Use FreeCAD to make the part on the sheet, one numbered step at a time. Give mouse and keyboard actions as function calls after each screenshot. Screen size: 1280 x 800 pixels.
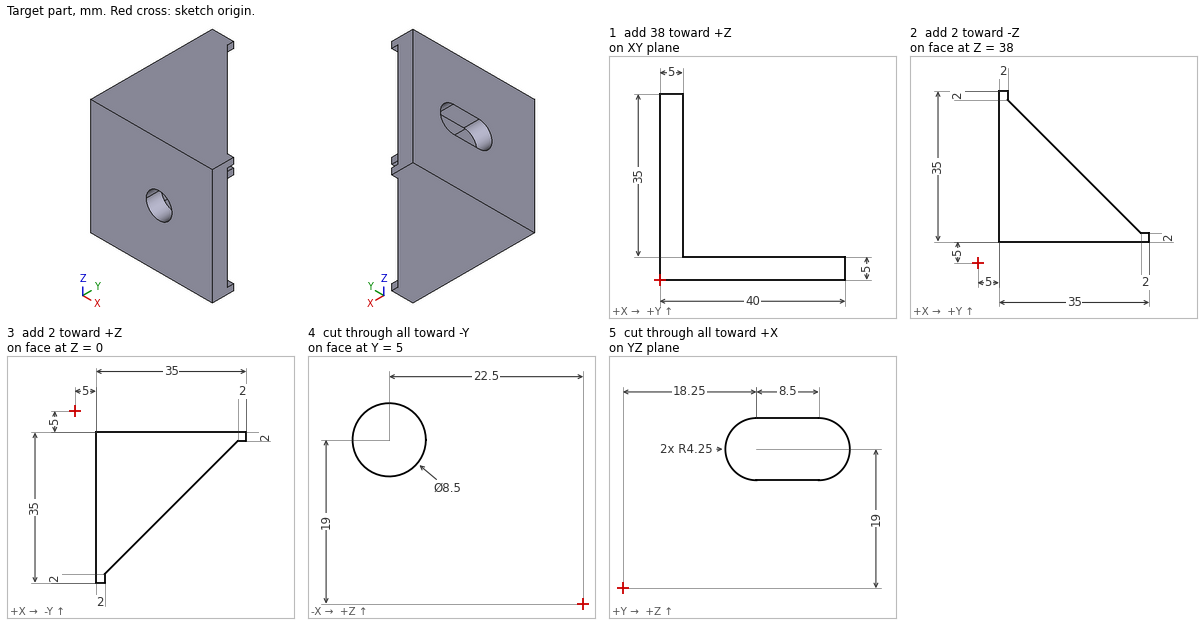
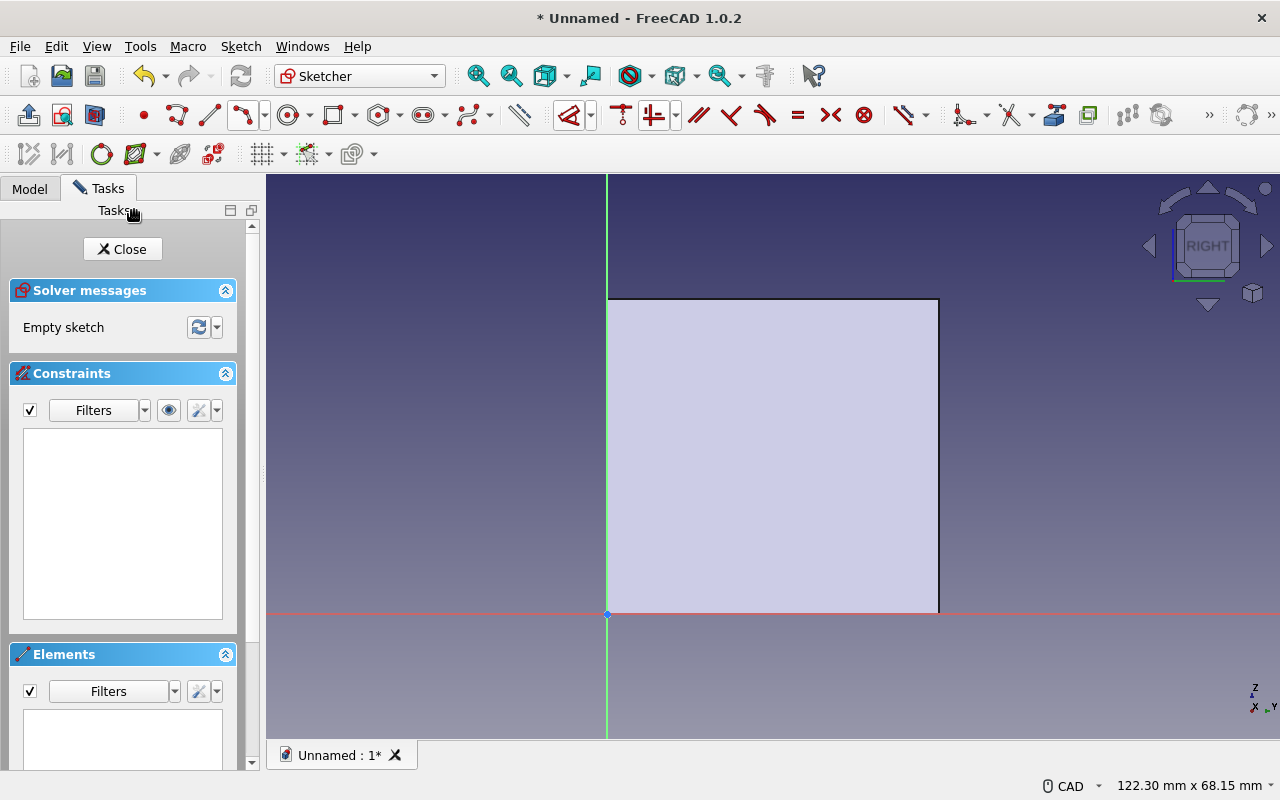
scroll(774, 592, up, 3)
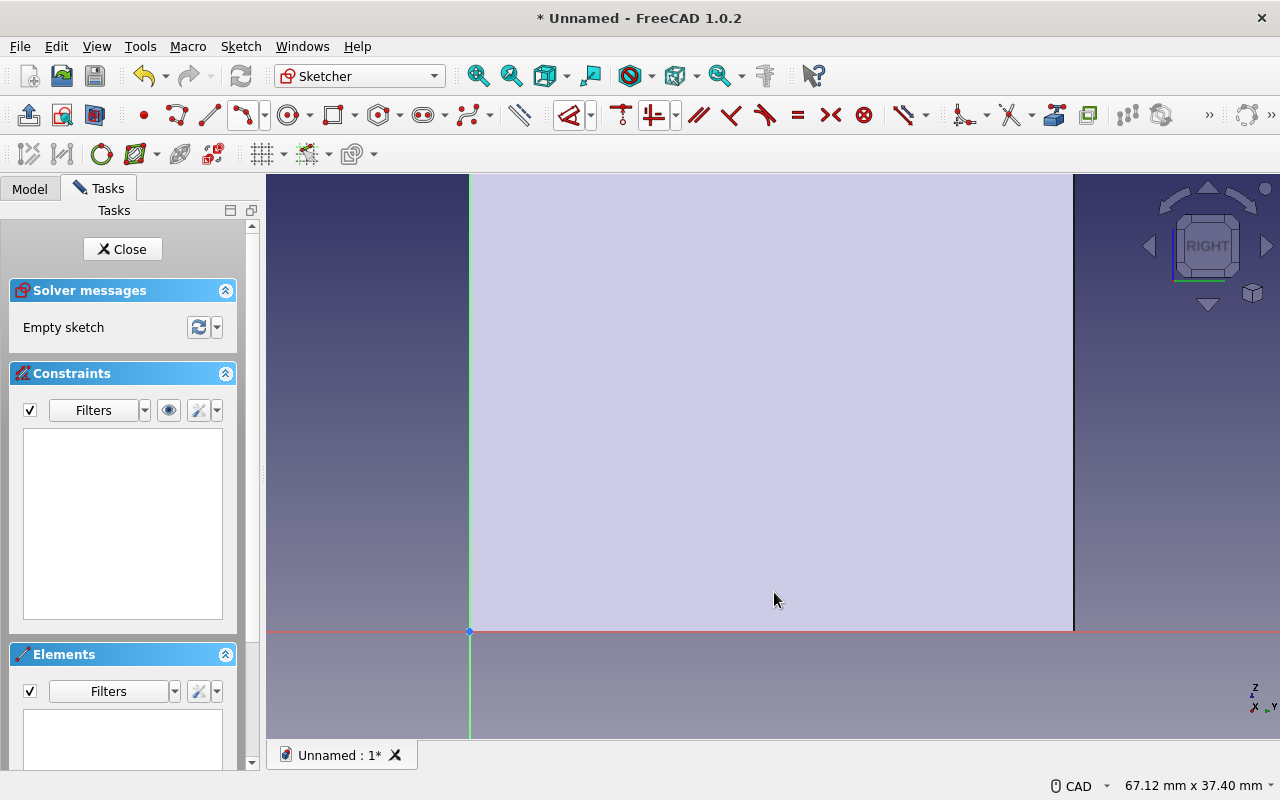
key(g)
key(s)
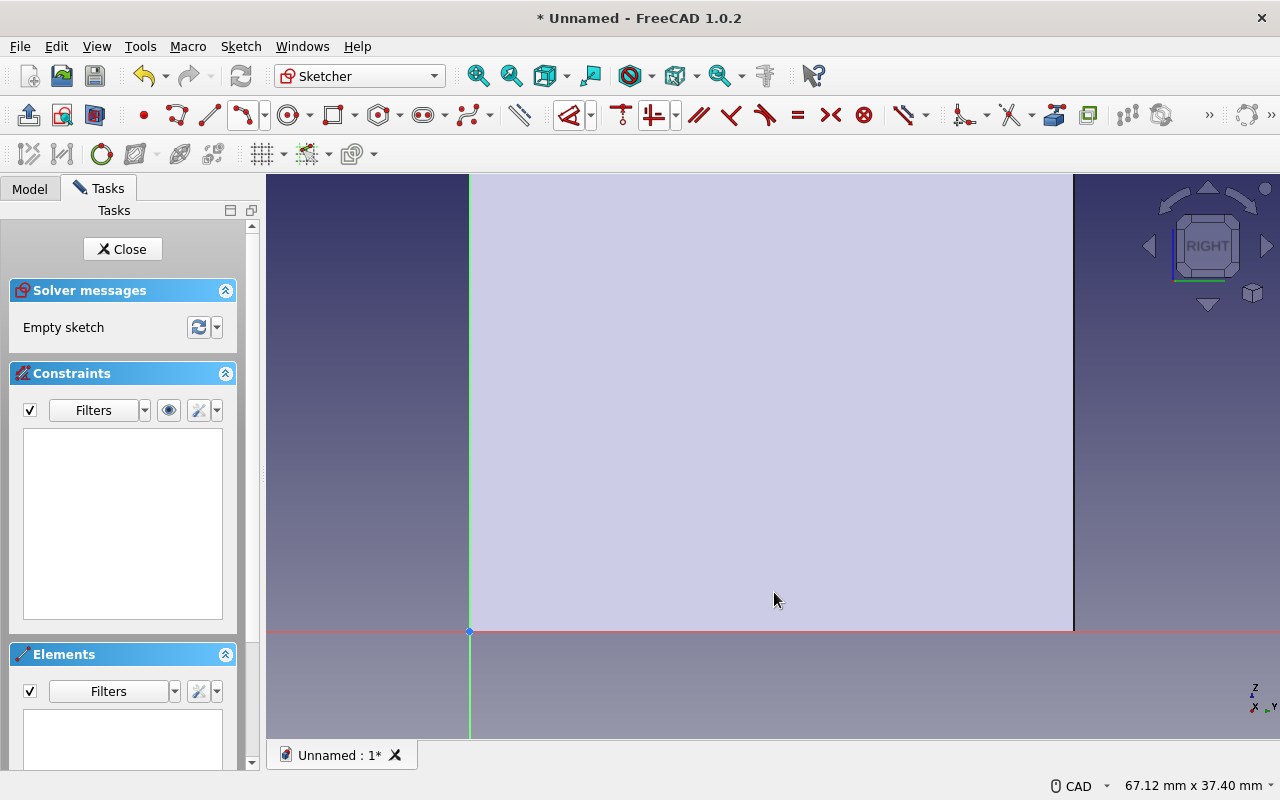
click(745, 344)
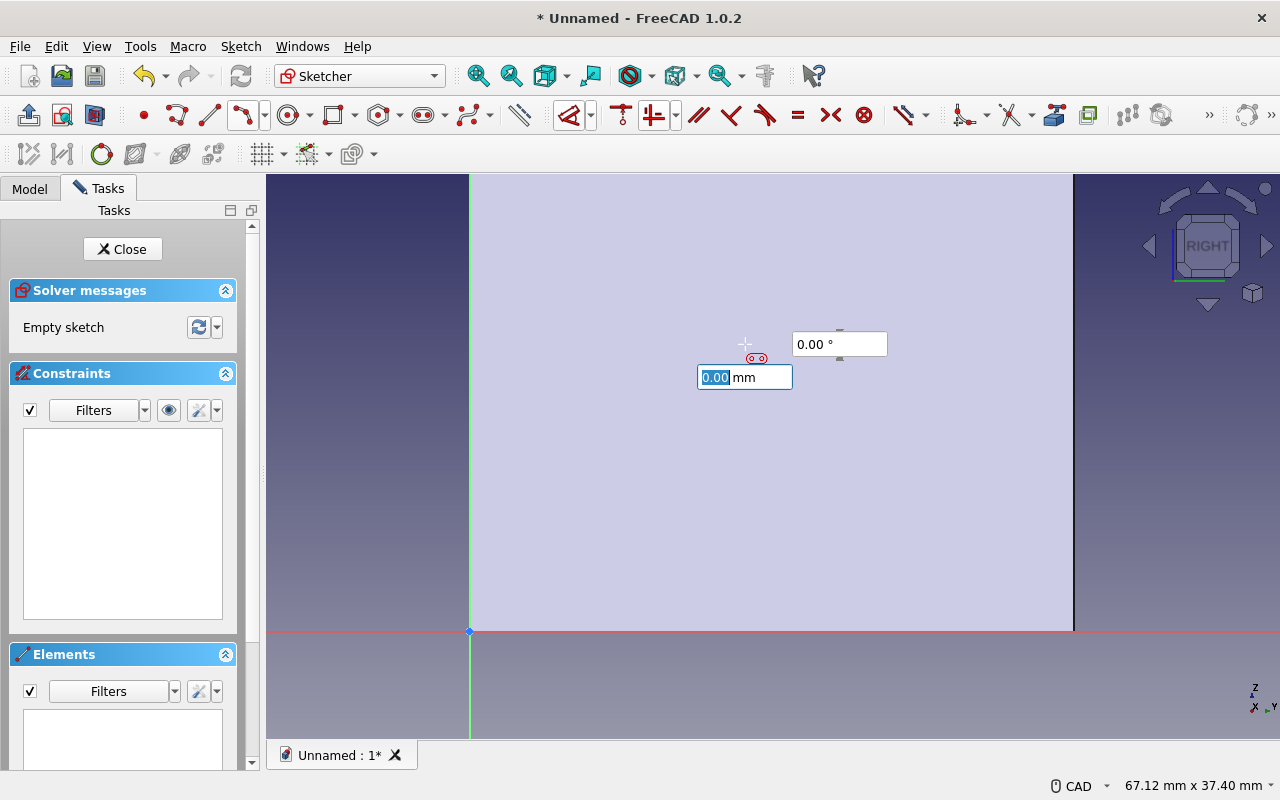
click(874, 344)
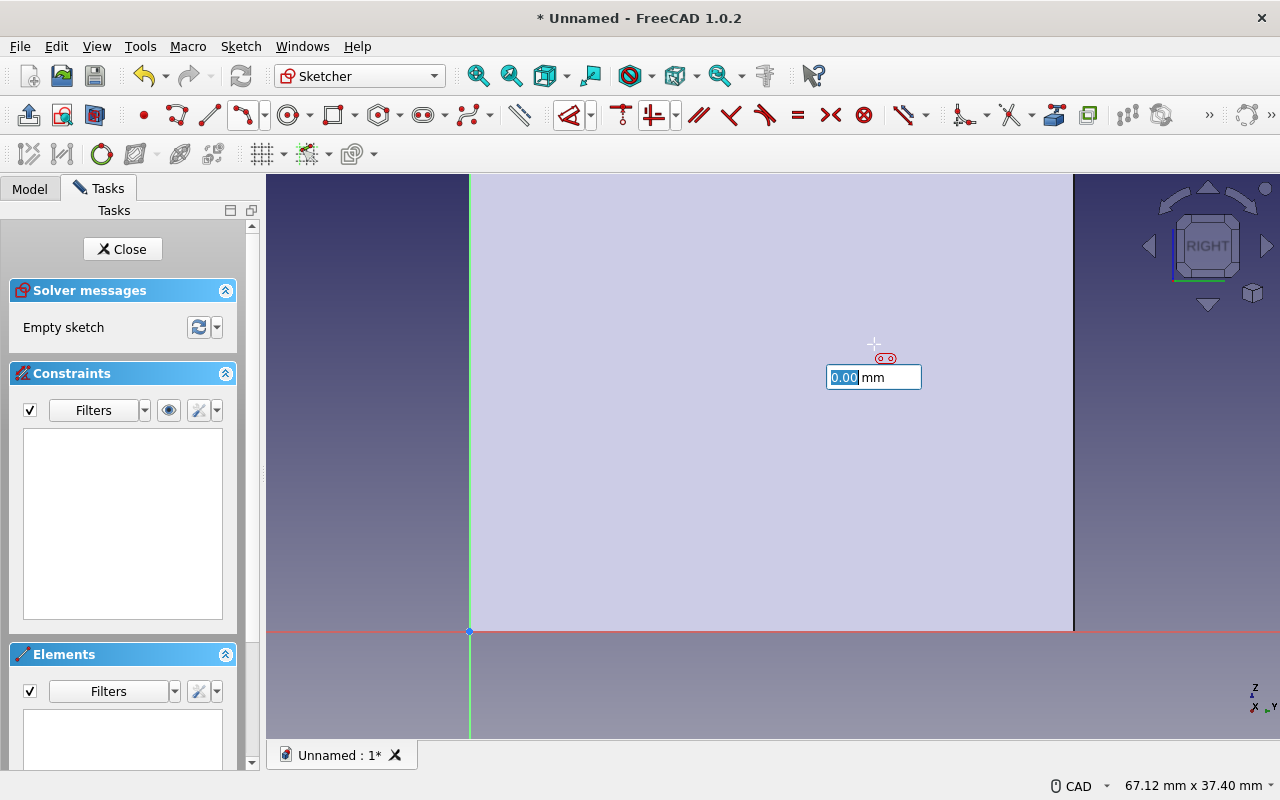
click(810, 280)
key(Escape)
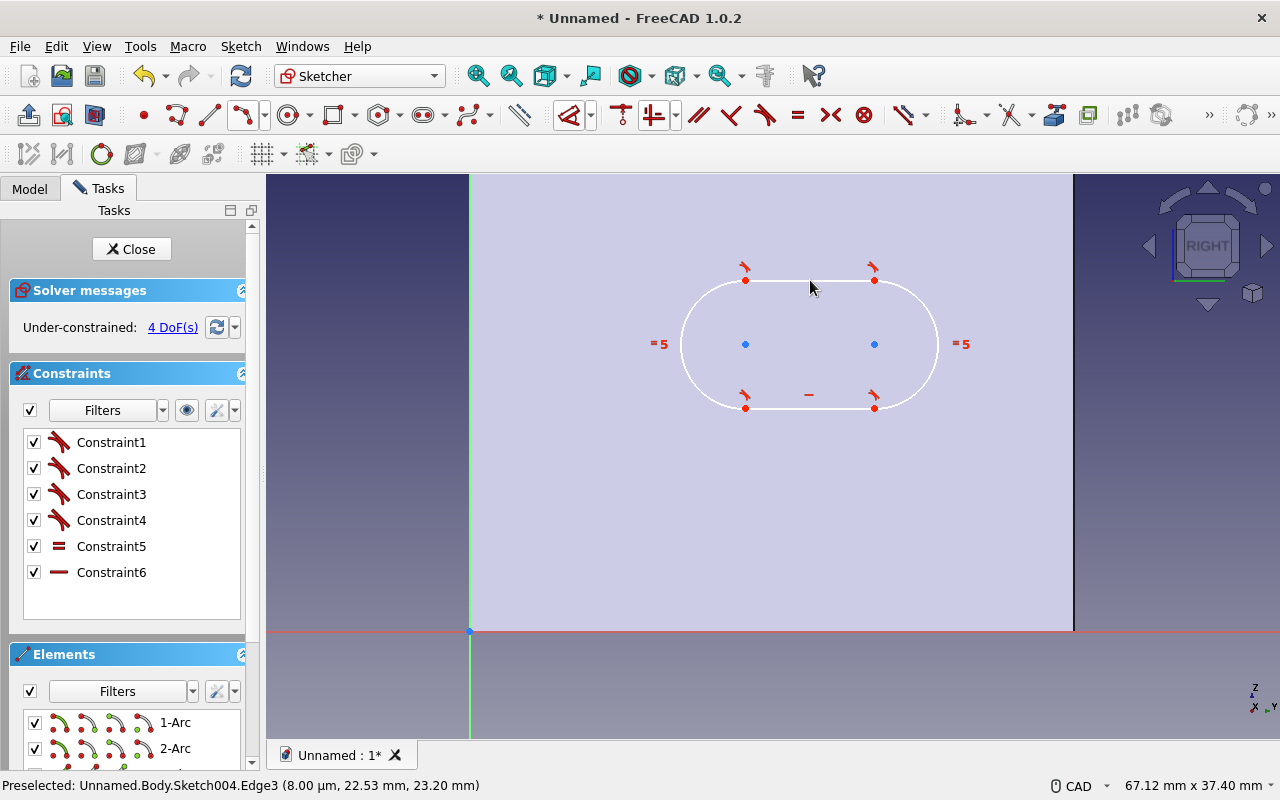
click(693, 307)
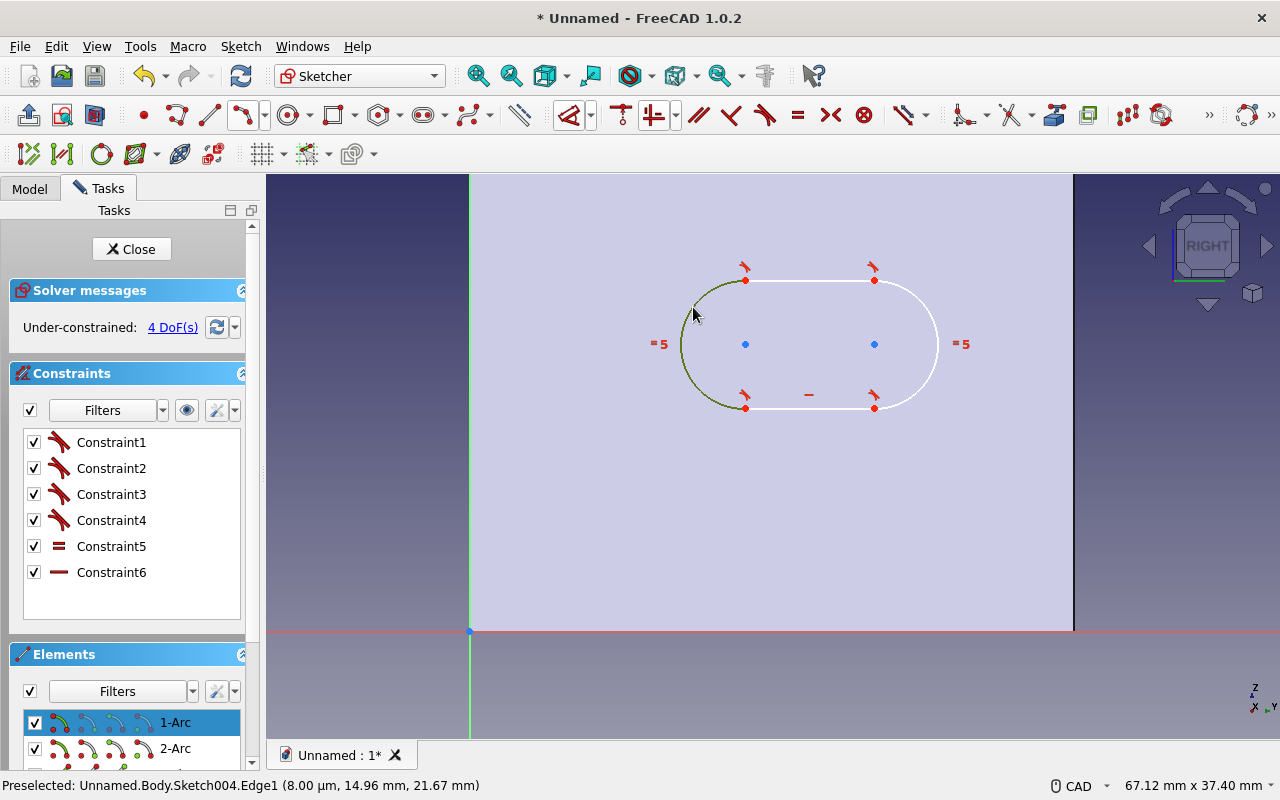
key(k)
key(r)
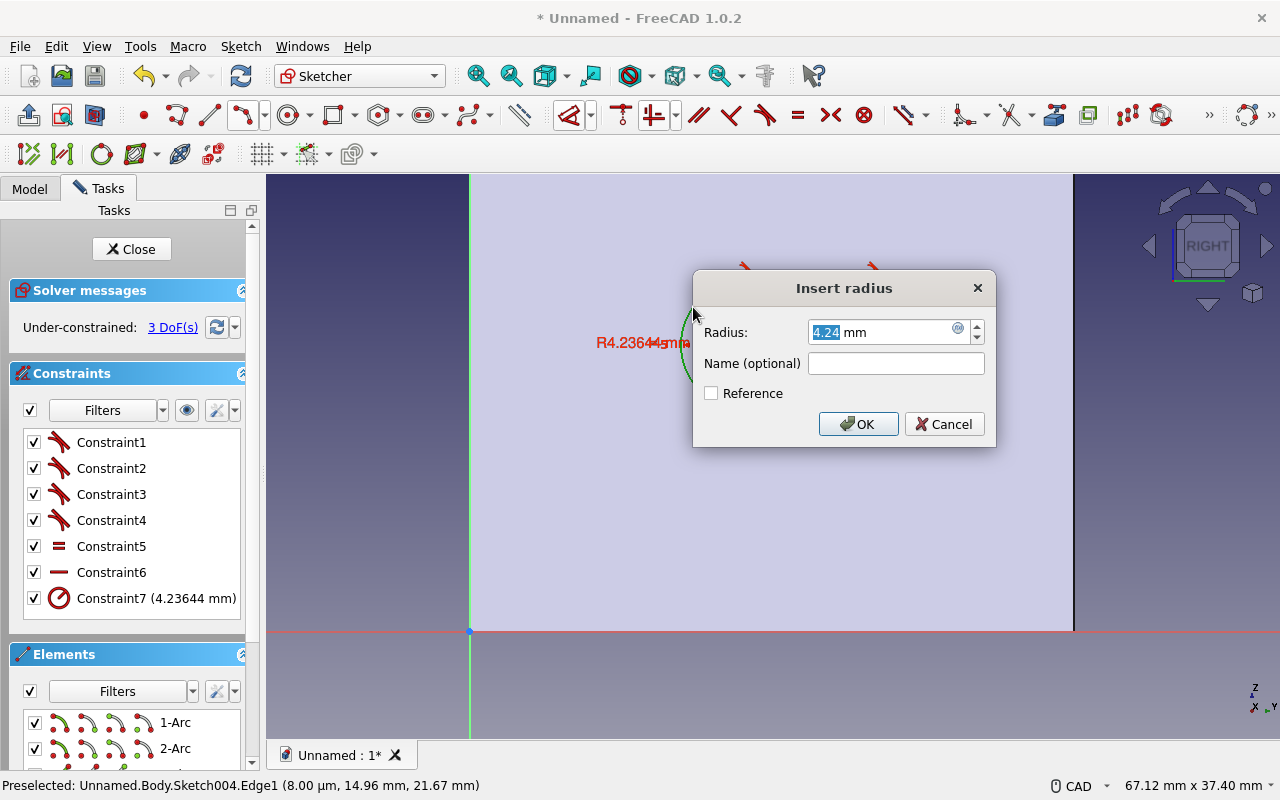
text(4.25)
key(Return)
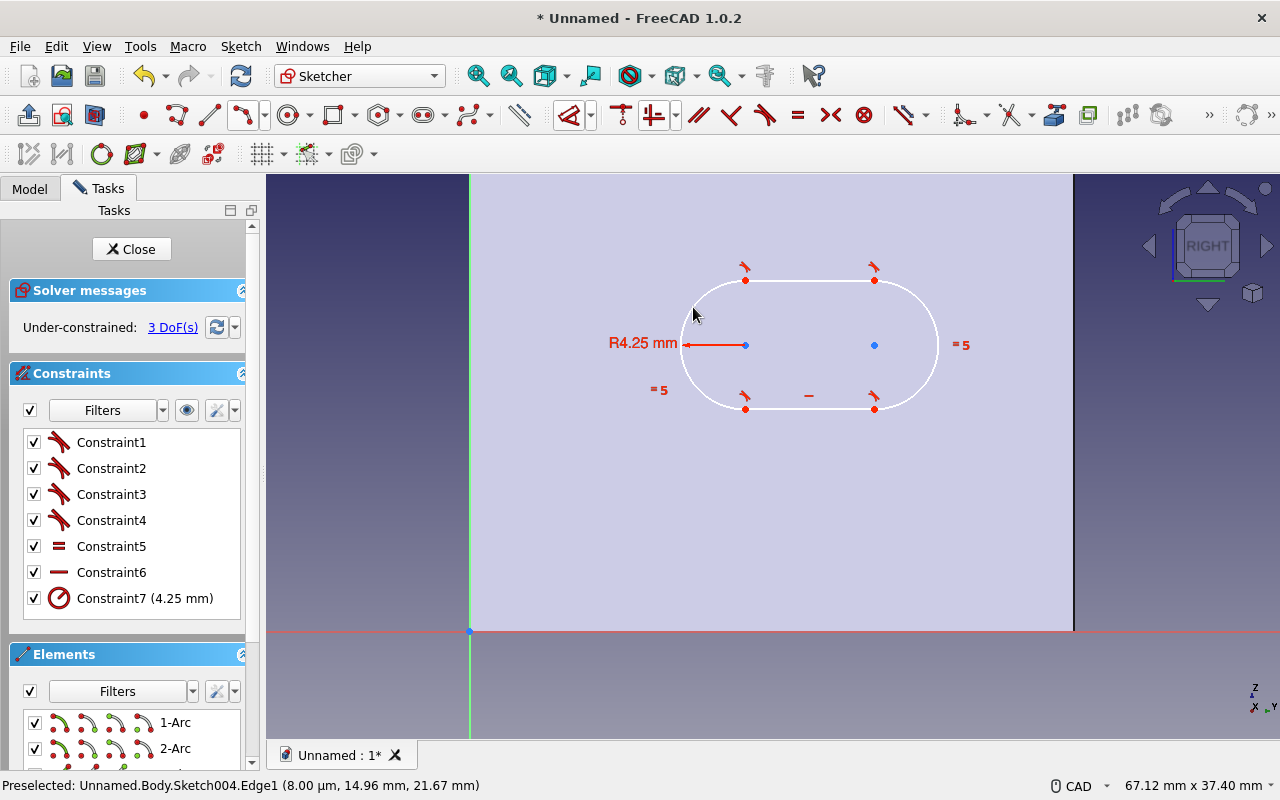
click(784, 281)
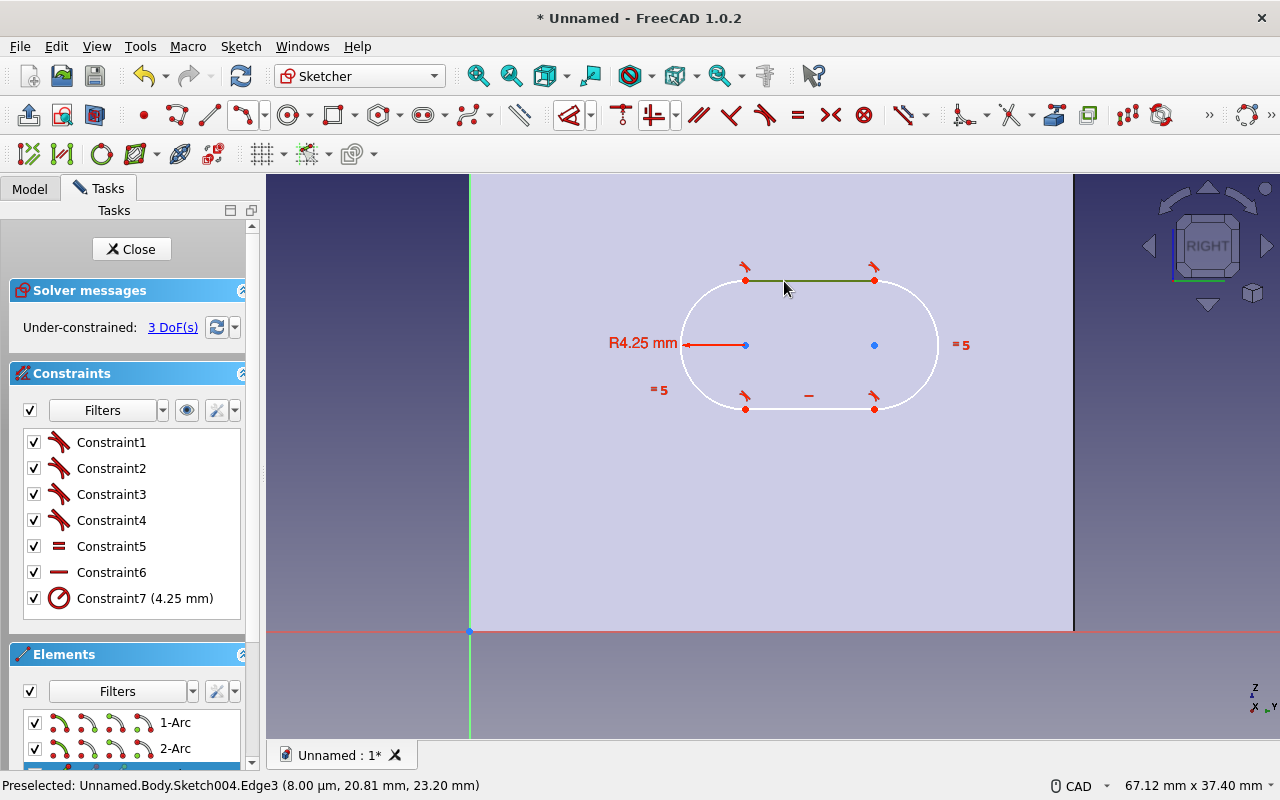
key(l)